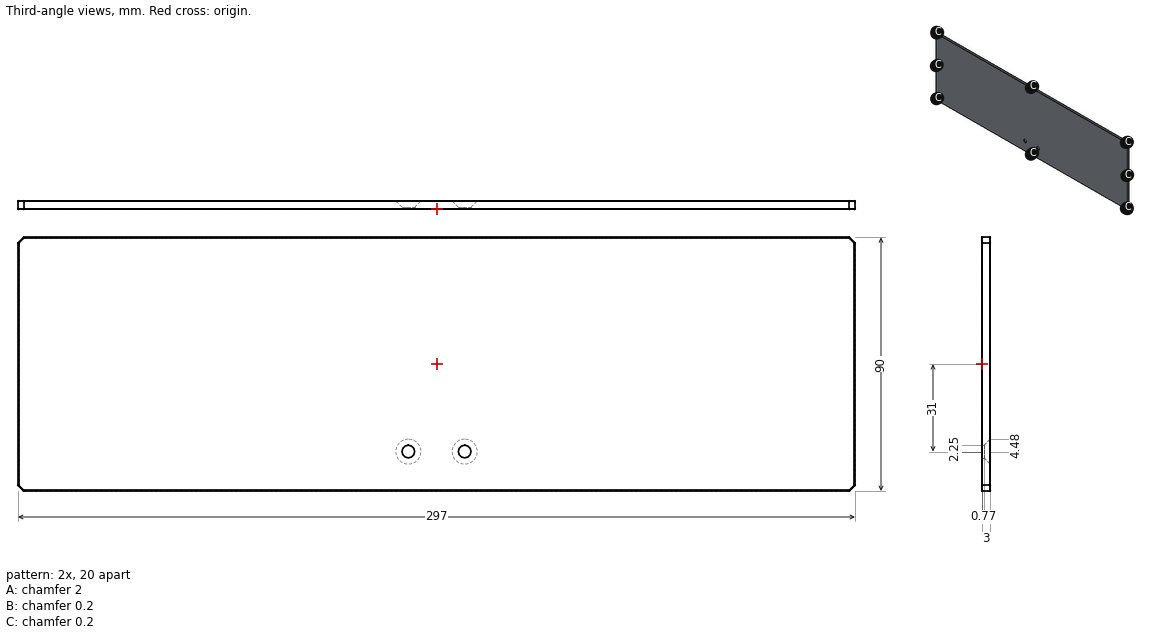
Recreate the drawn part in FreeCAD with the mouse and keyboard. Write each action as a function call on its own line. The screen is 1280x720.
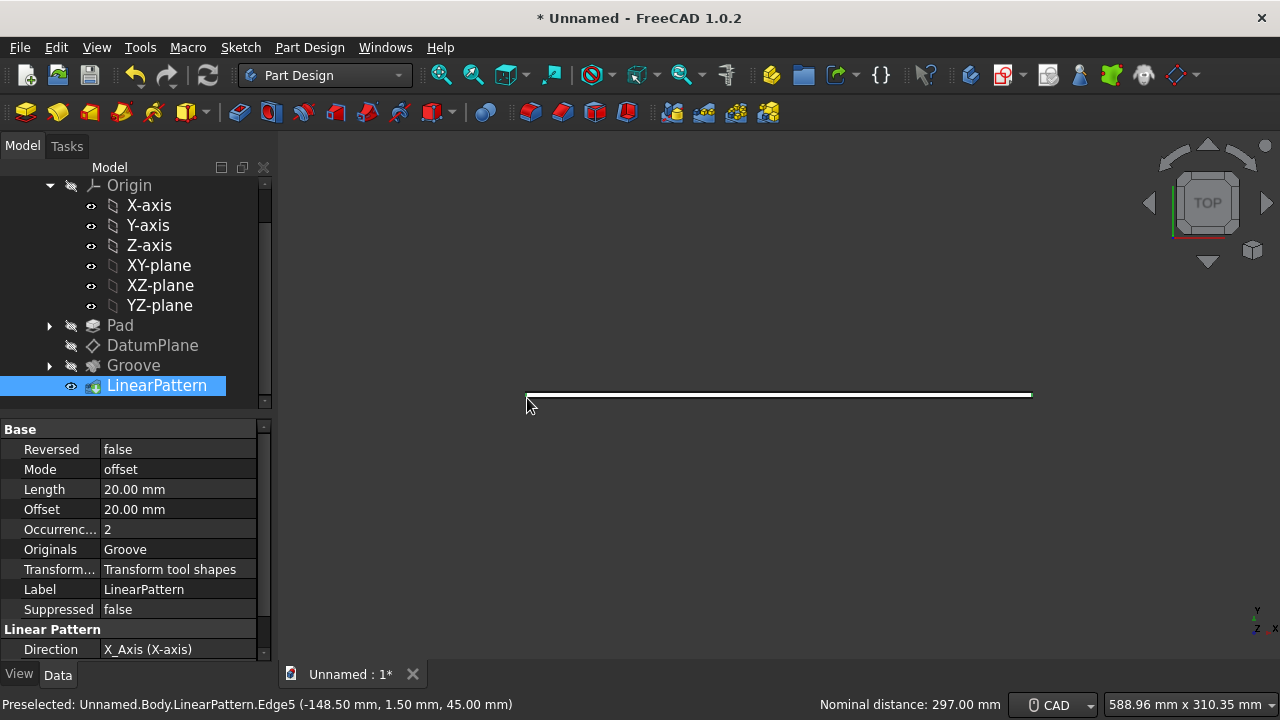
key(1)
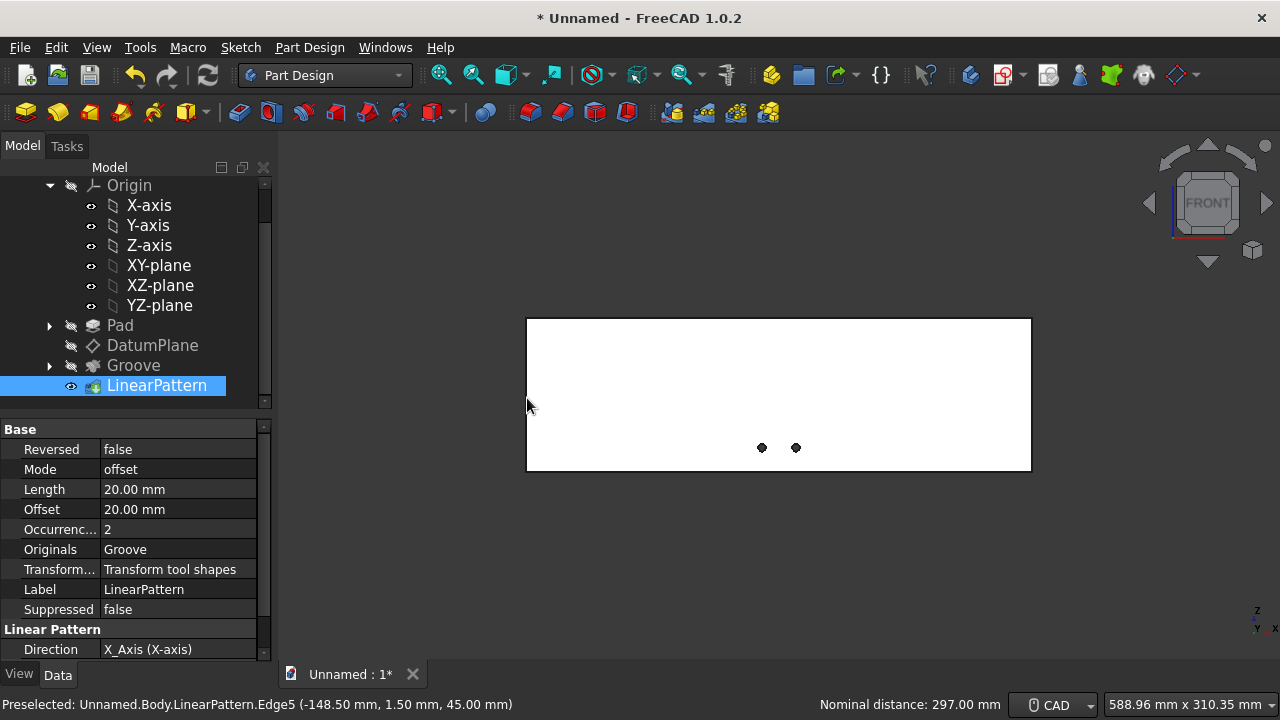
scroll(526, 471, up, 11)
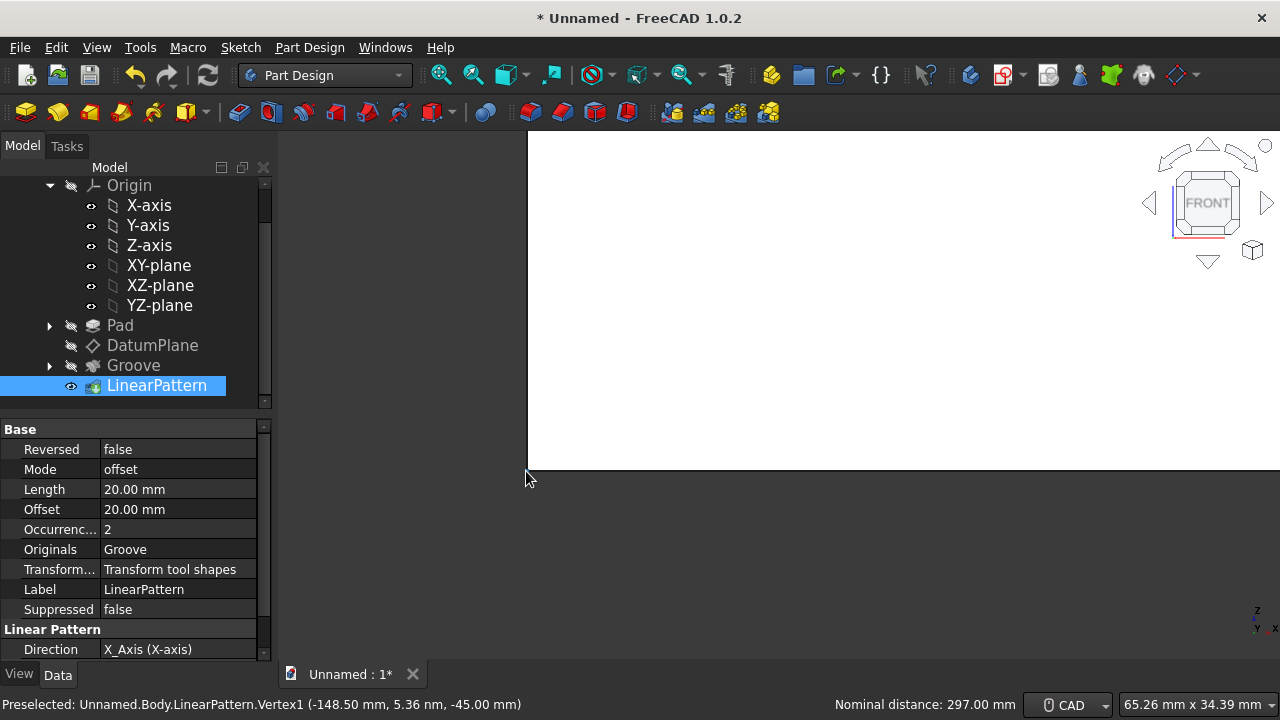
key(v)
key(f)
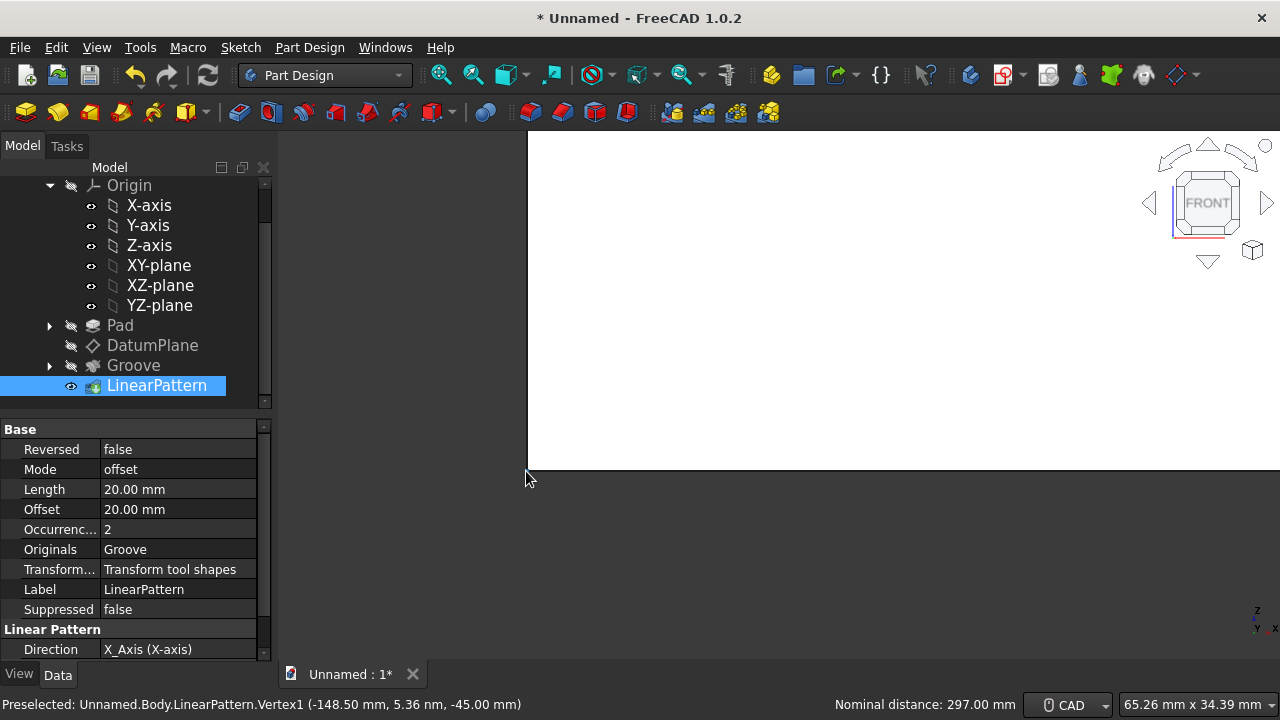
key(3)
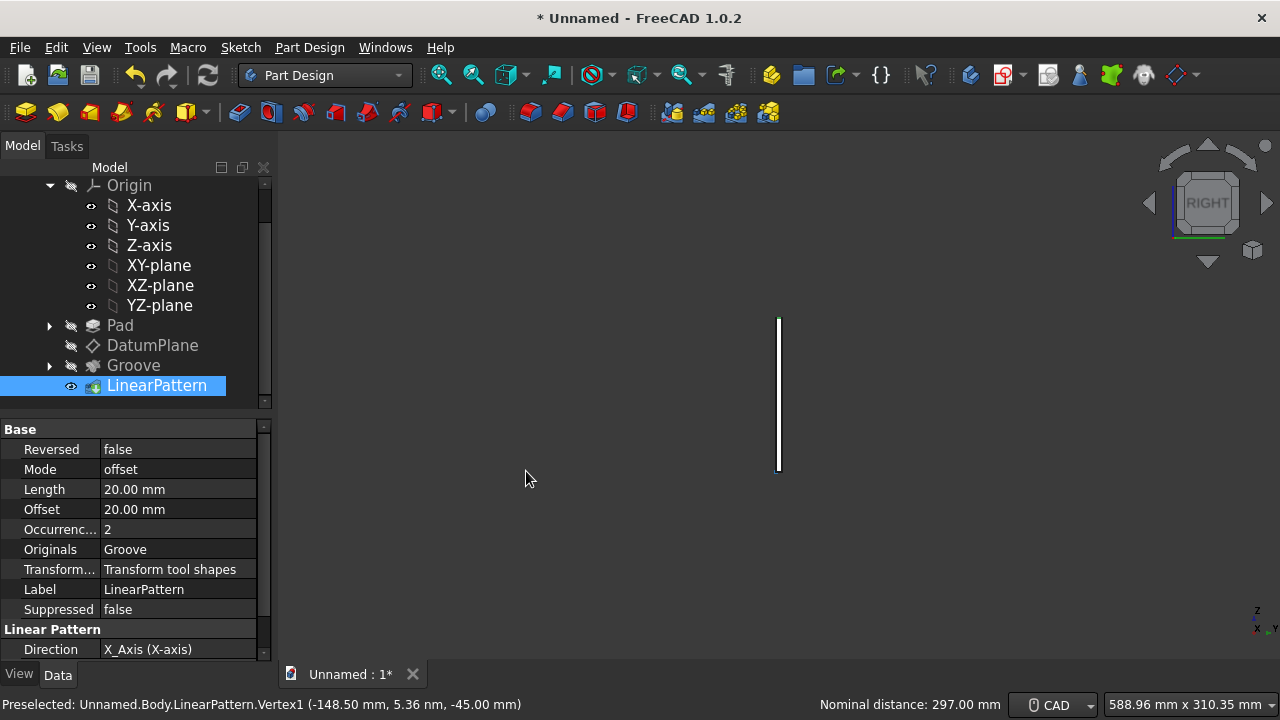
click(442, 76)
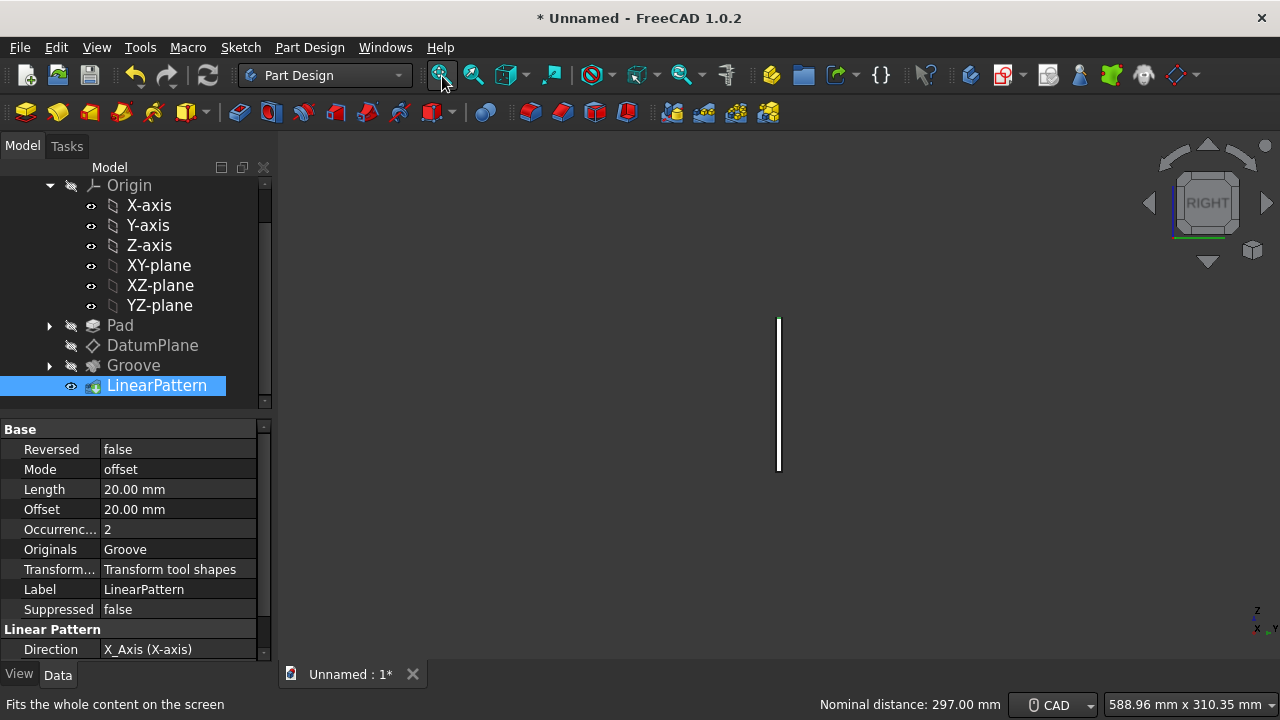
scroll(779, 471, up, 11)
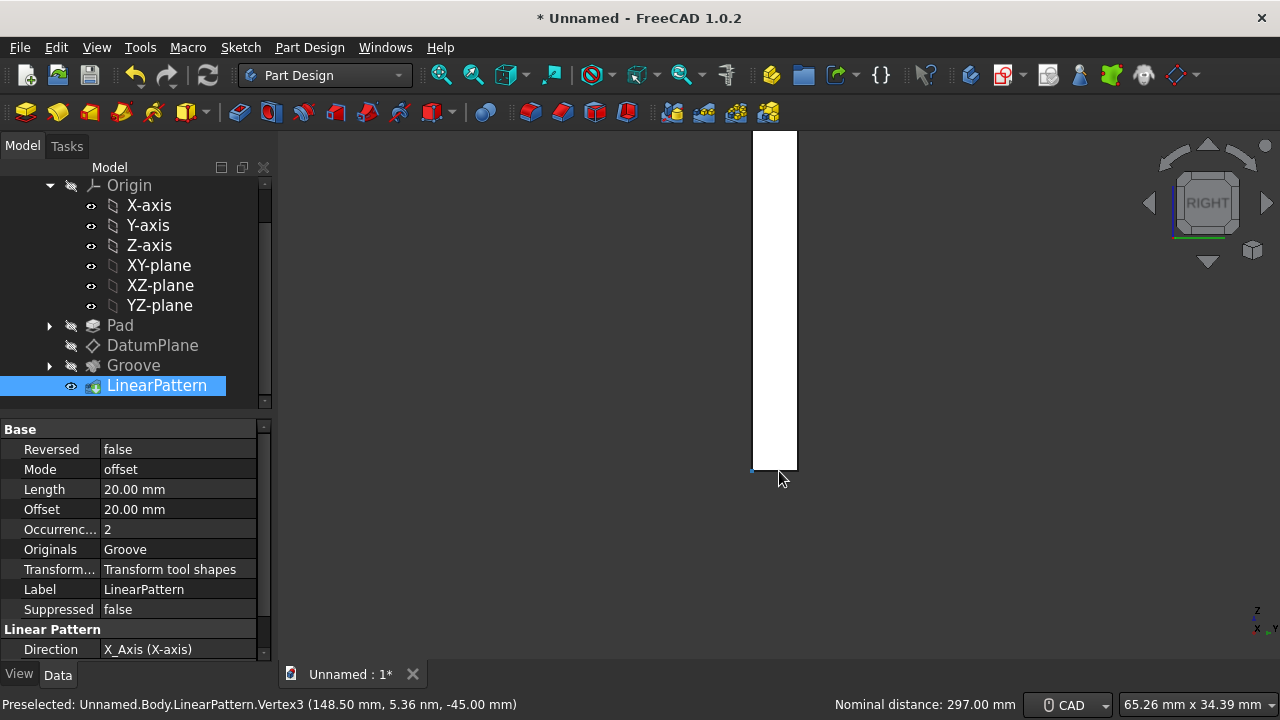
click(775, 470, ctrl)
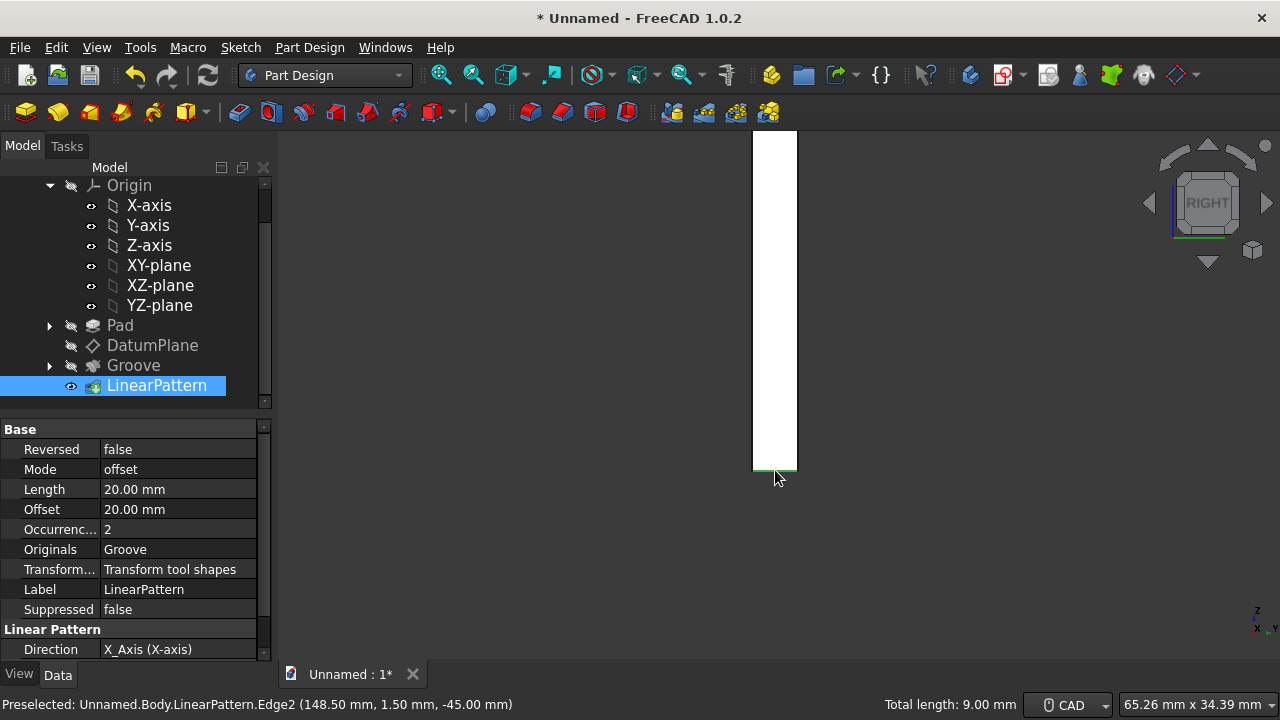
key(v)
key(f)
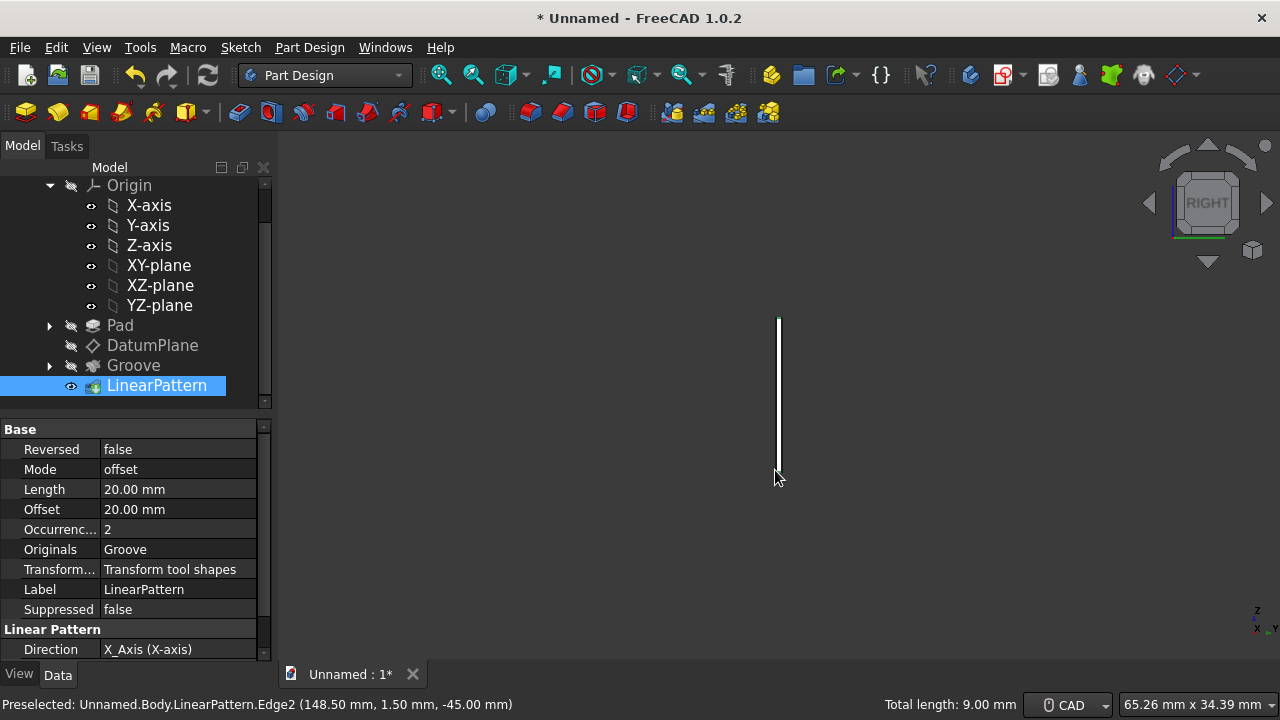
key(5)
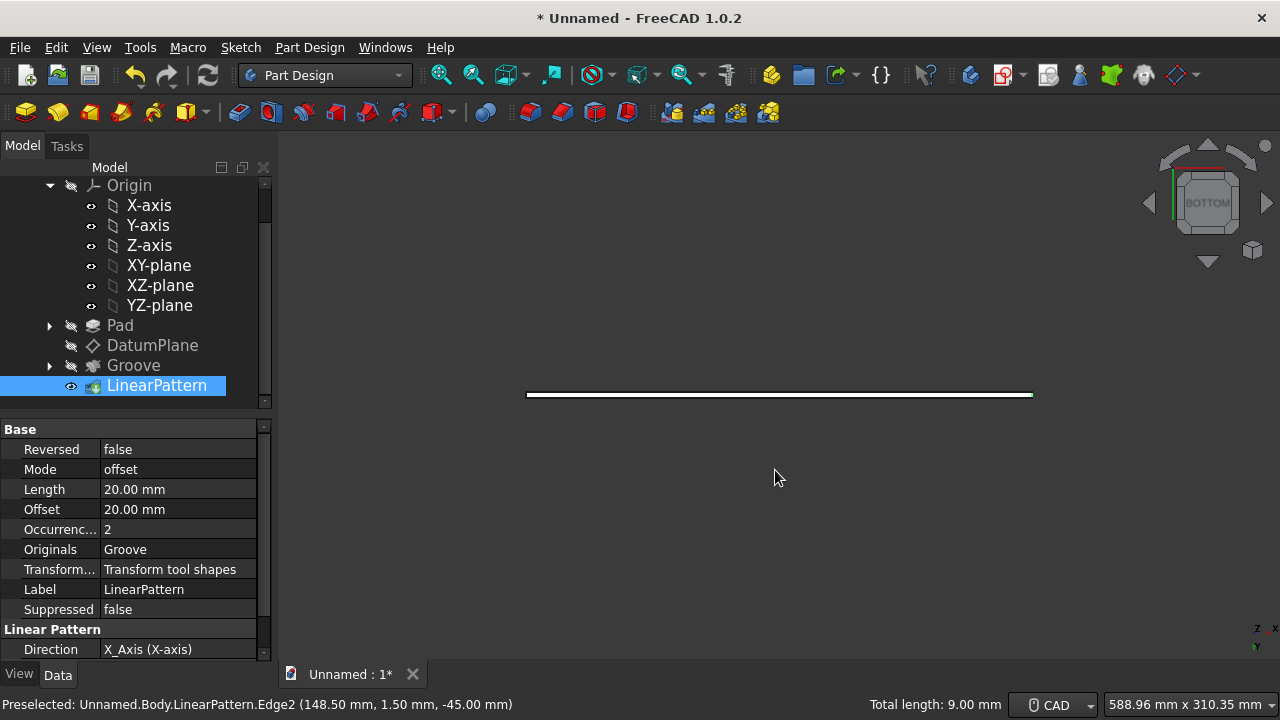
scroll(526, 394, up, 11)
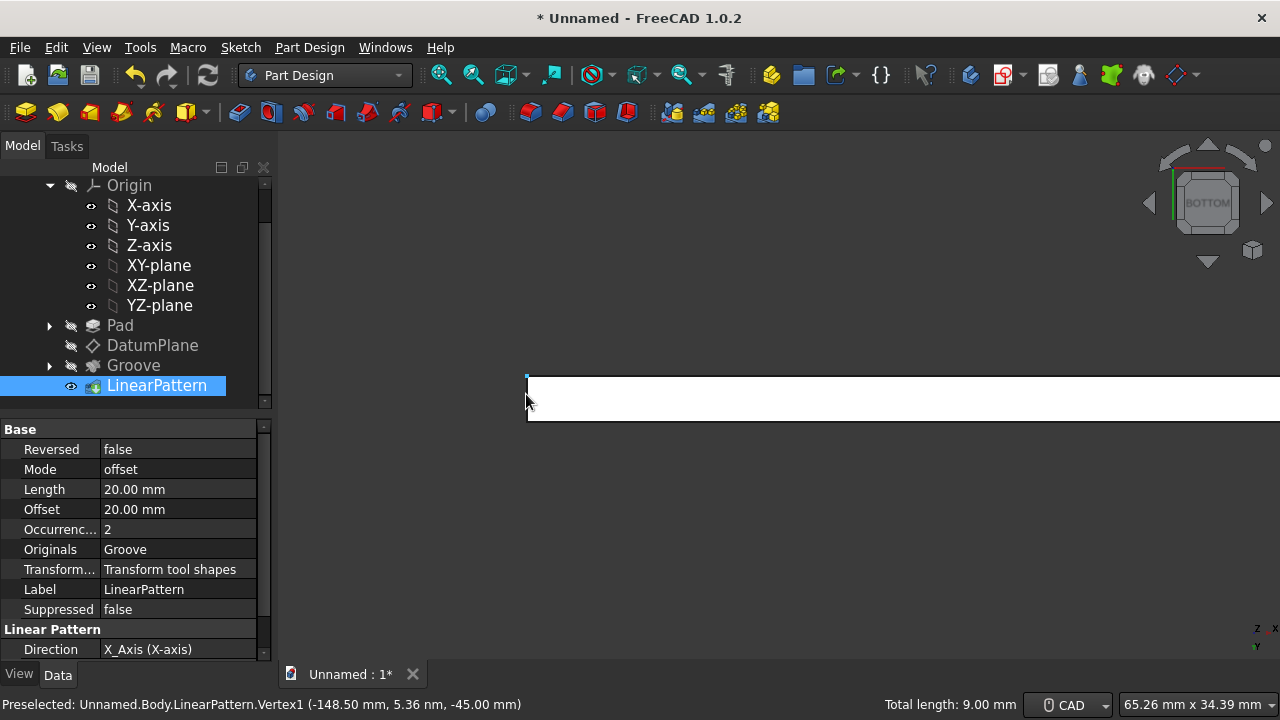
click(527, 398, ctrl)